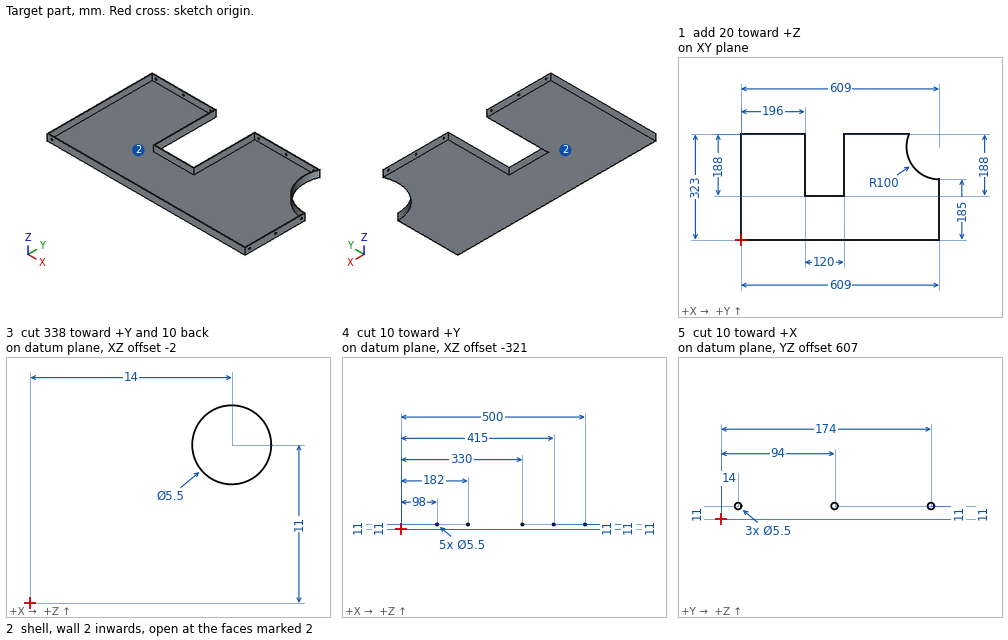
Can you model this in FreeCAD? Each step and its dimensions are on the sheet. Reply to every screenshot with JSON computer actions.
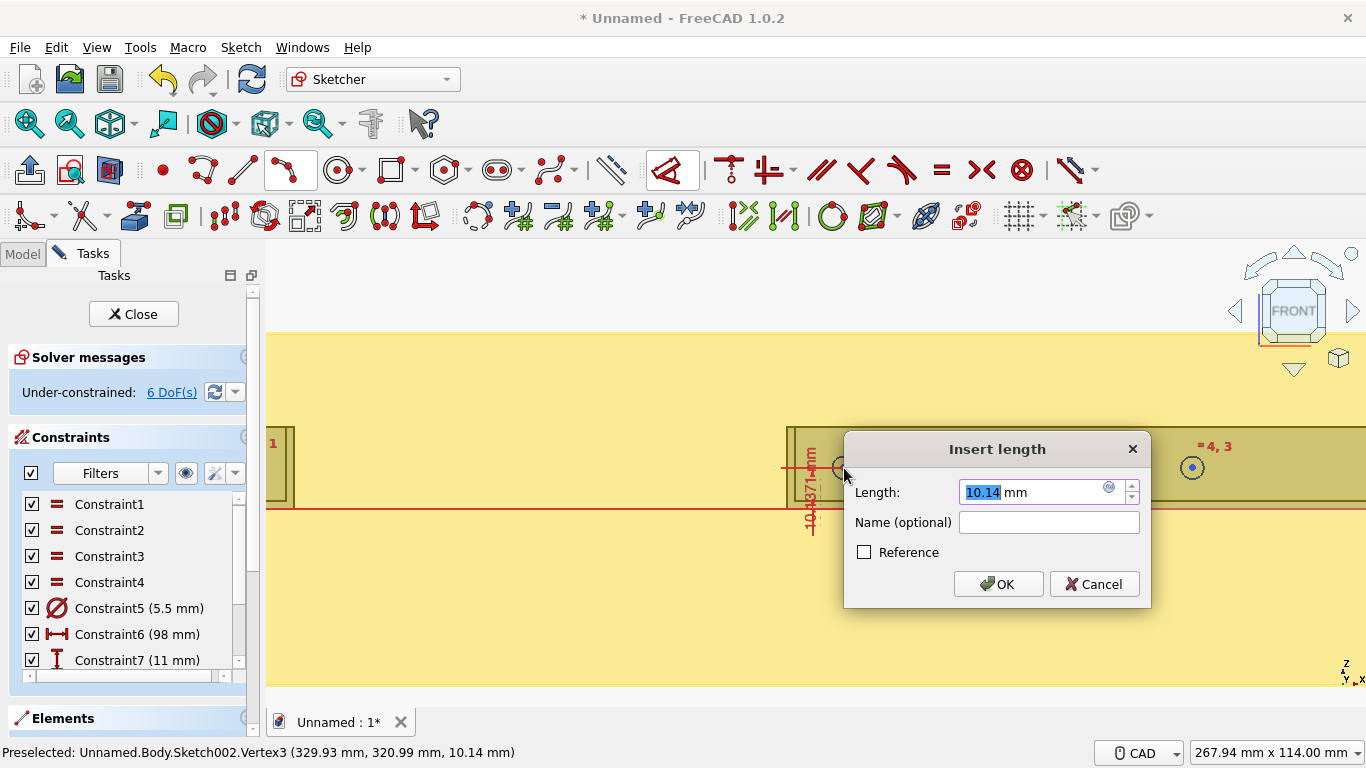
{"action": "type", "text": "11"}
{"action": "key", "text": "Return"}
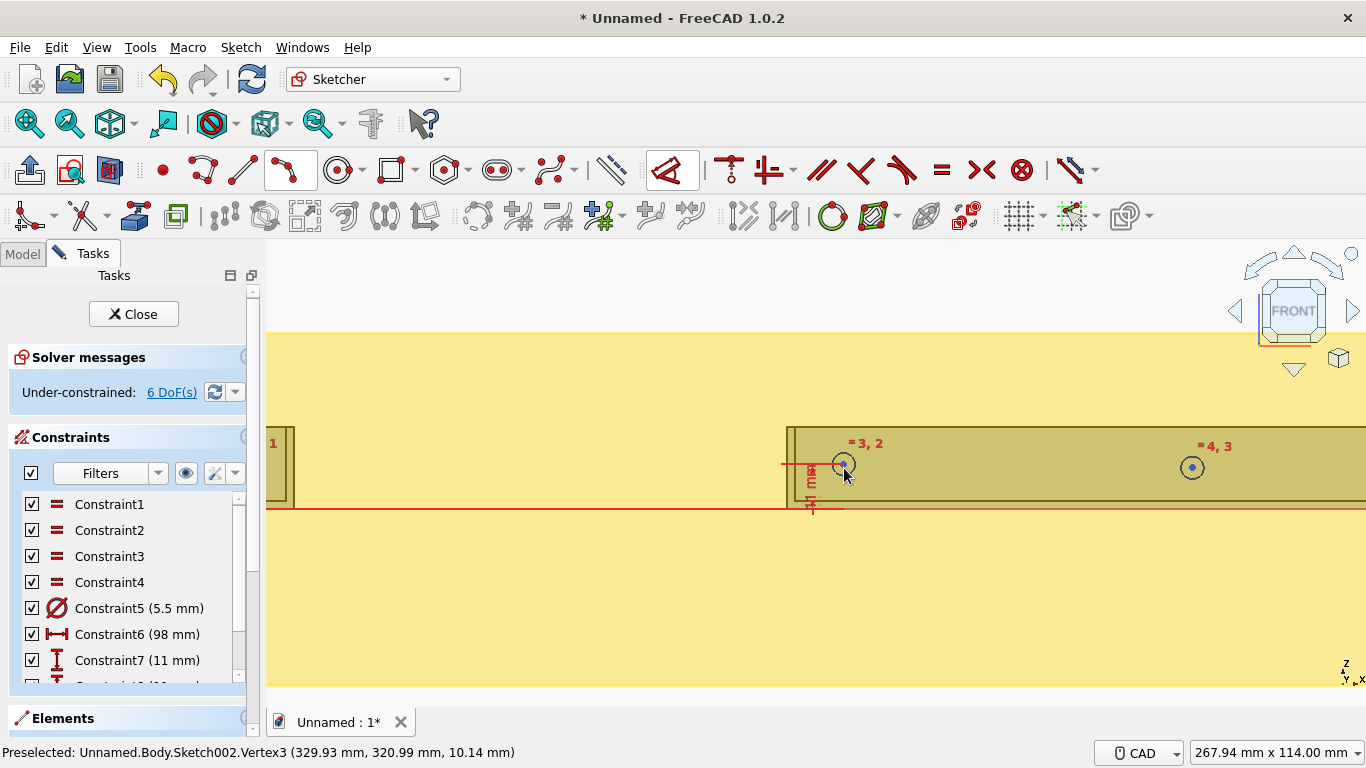
{"action": "left_click", "coordinate": [1192, 468]}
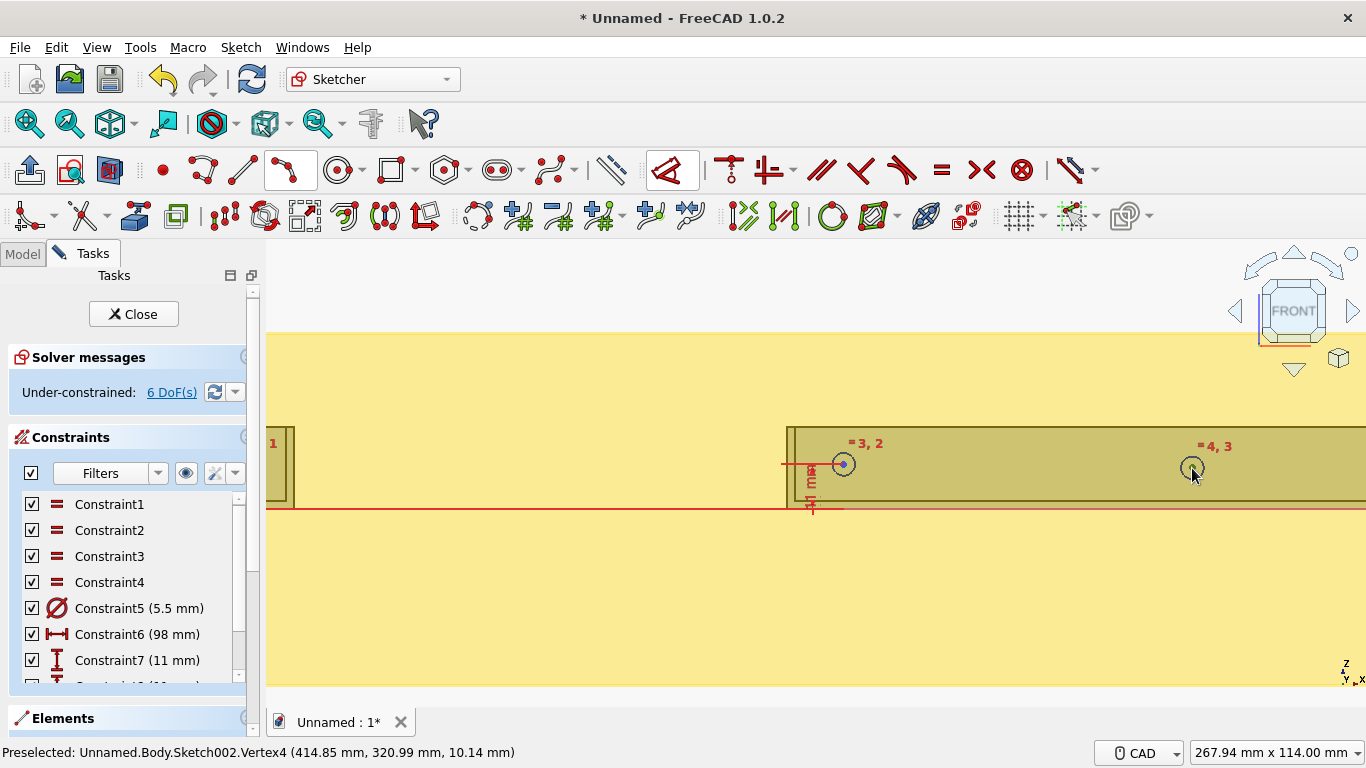
{"action": "key", "text": "i"}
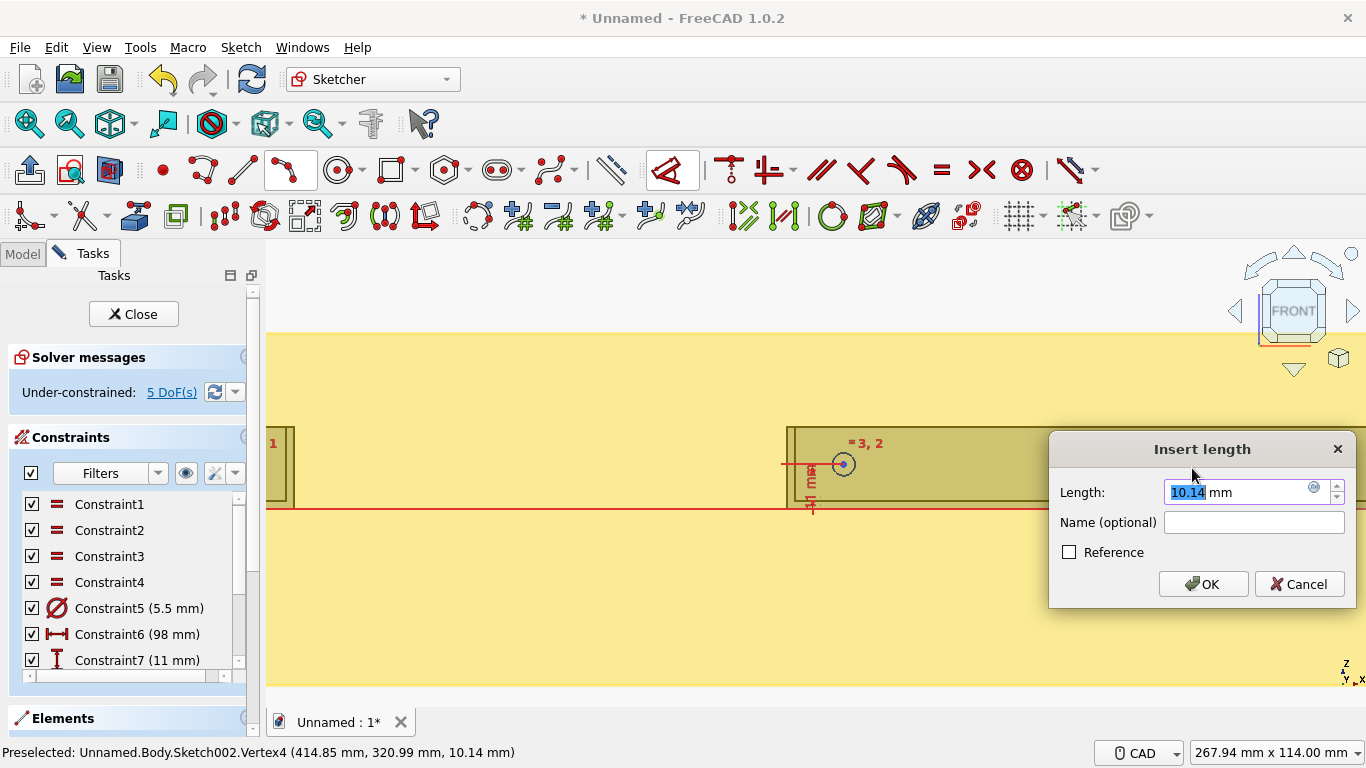
{"action": "type", "text": "11"}
{"action": "key", "text": "Return"}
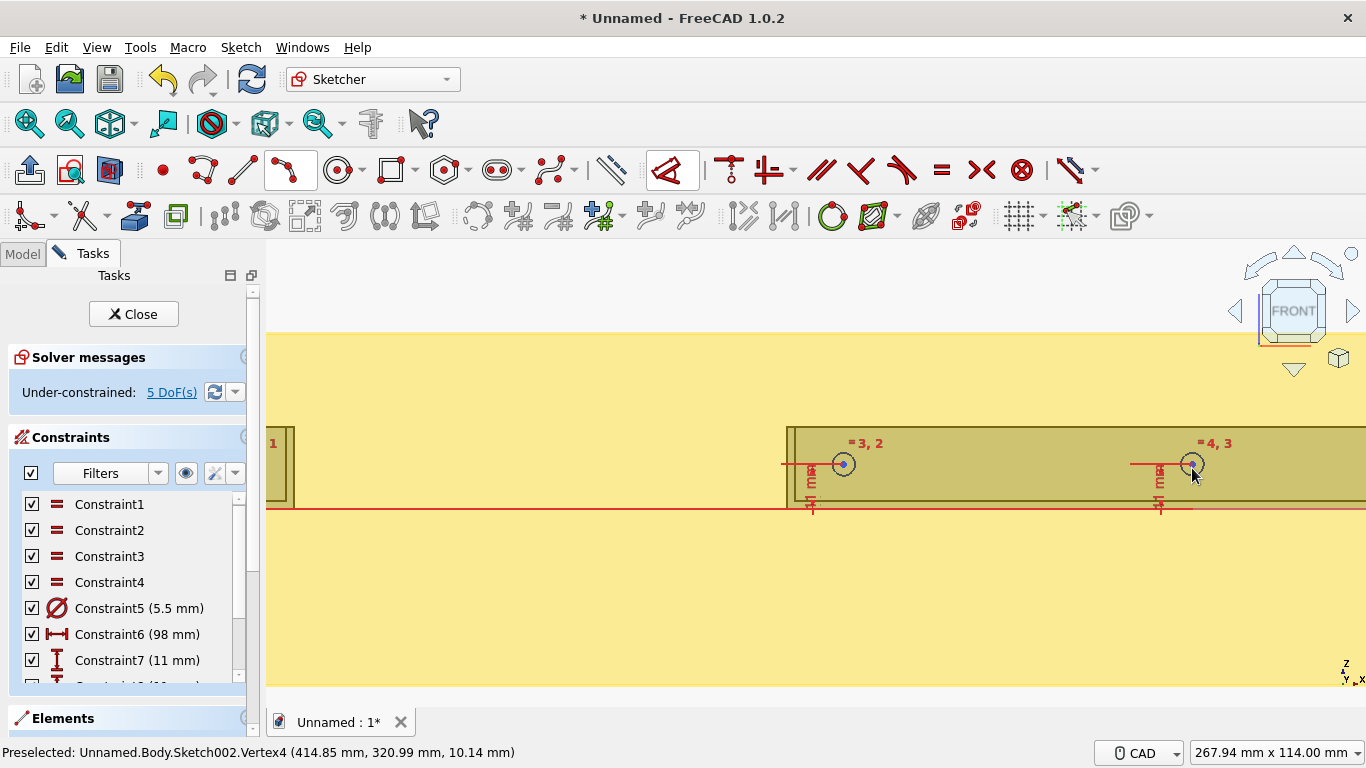
{"action": "scroll", "coordinate": [845, 469], "scroll_direction": "down", "scroll_amount": 6}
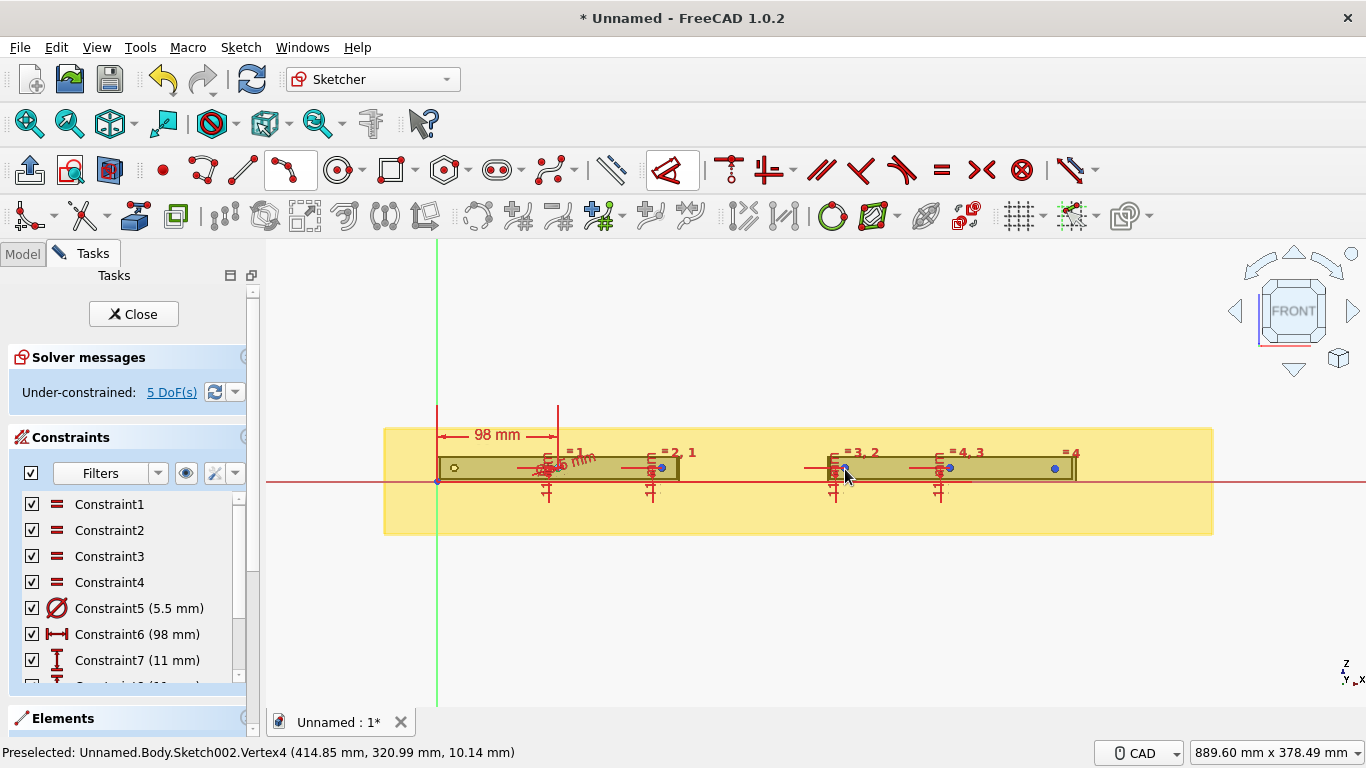
{"action": "scroll", "coordinate": [1055, 469], "scroll_direction": "up", "scroll_amount": 6}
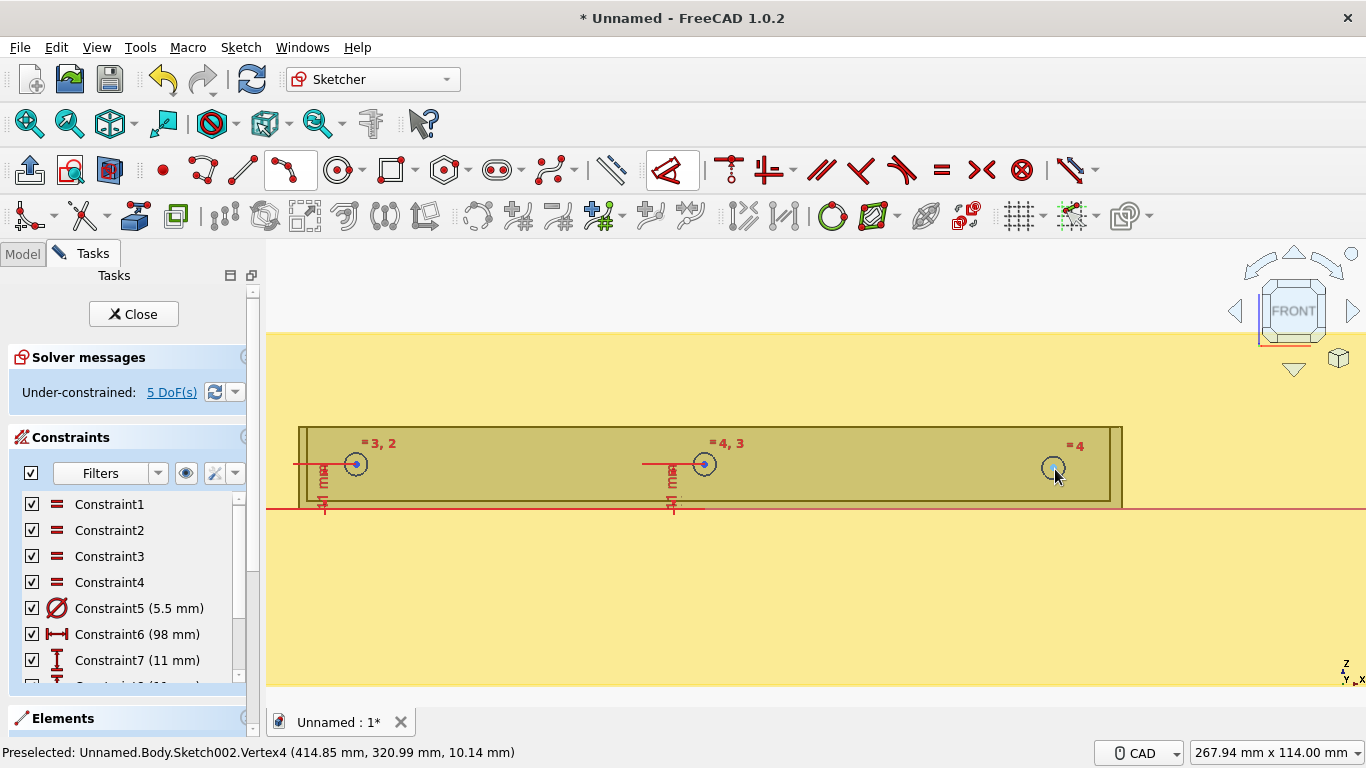
{"action": "left_click", "coordinate": [1053, 468]}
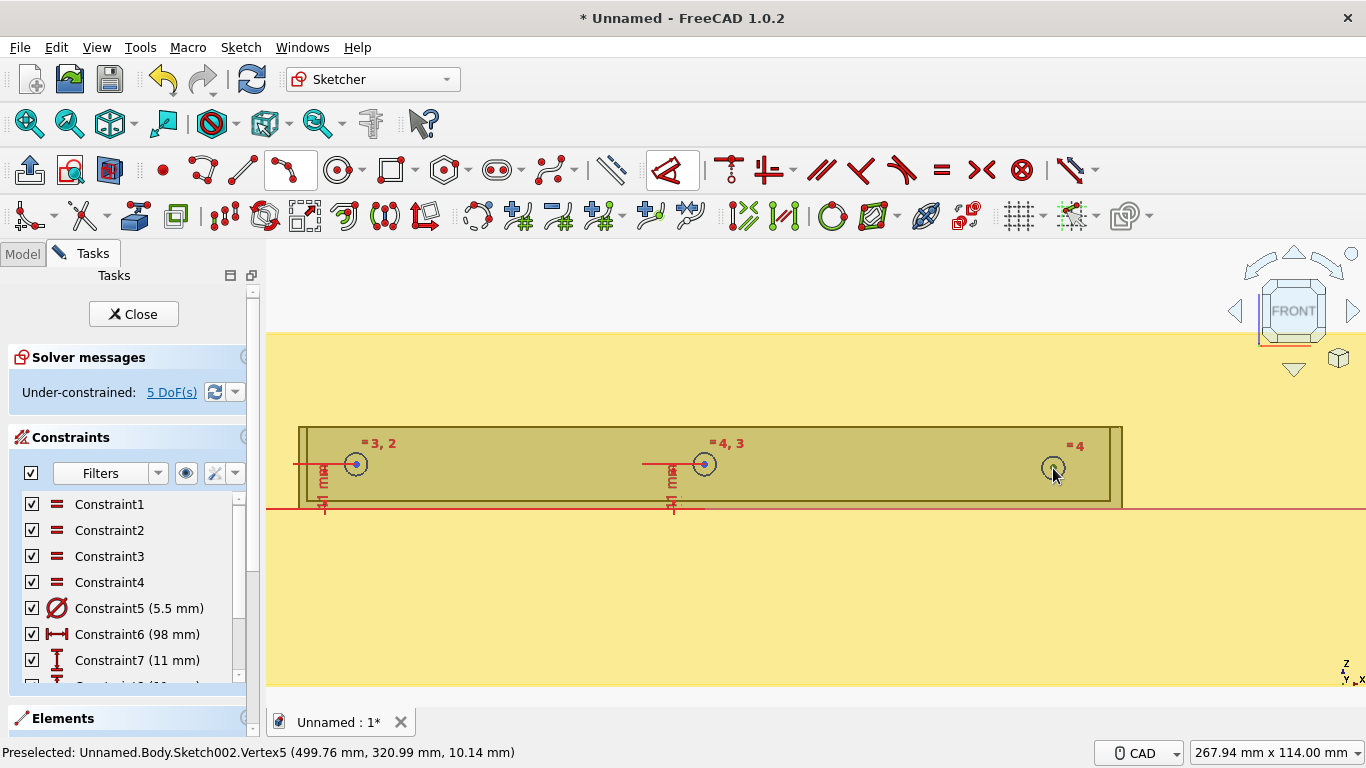
{"action": "key", "text": "i"}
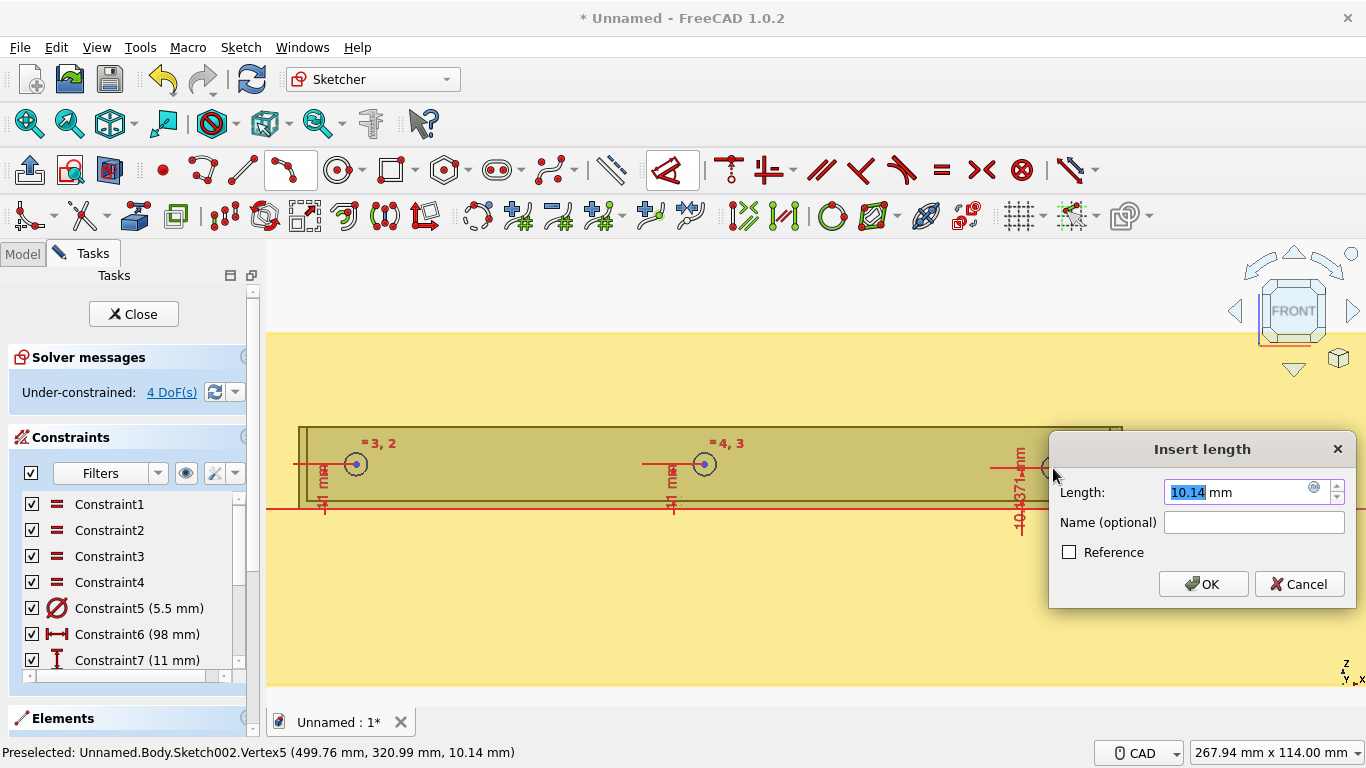
{"action": "type", "text": "11"}
{"action": "key", "text": "Return"}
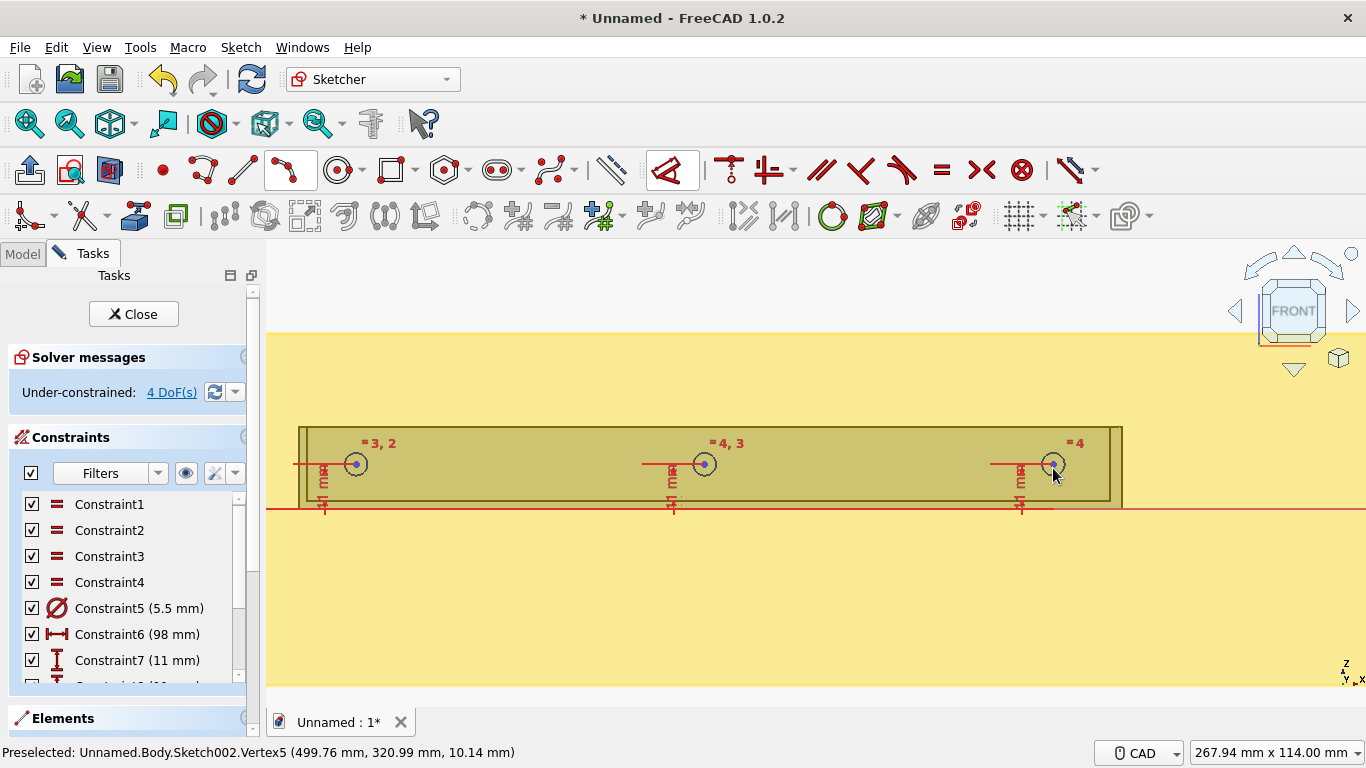
{"action": "scroll", "coordinate": [1055, 469], "scroll_direction": "down", "scroll_amount": 6}